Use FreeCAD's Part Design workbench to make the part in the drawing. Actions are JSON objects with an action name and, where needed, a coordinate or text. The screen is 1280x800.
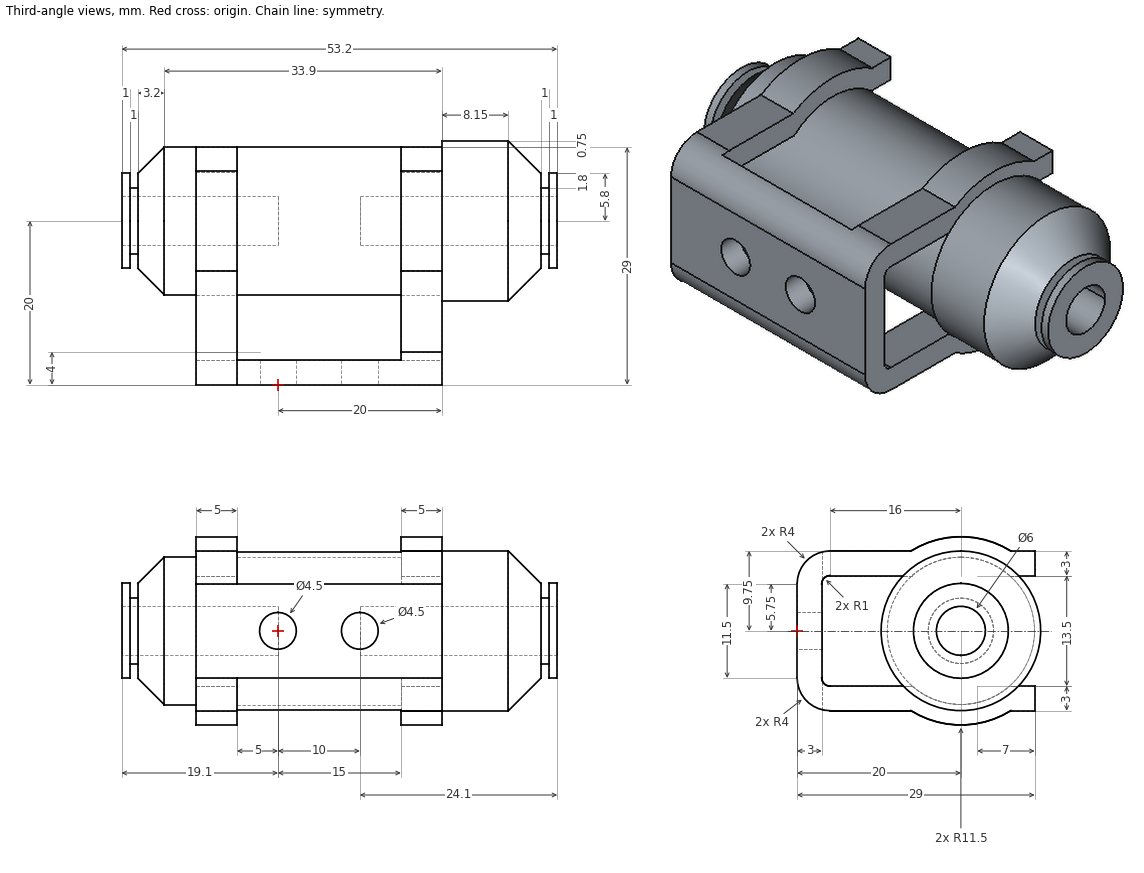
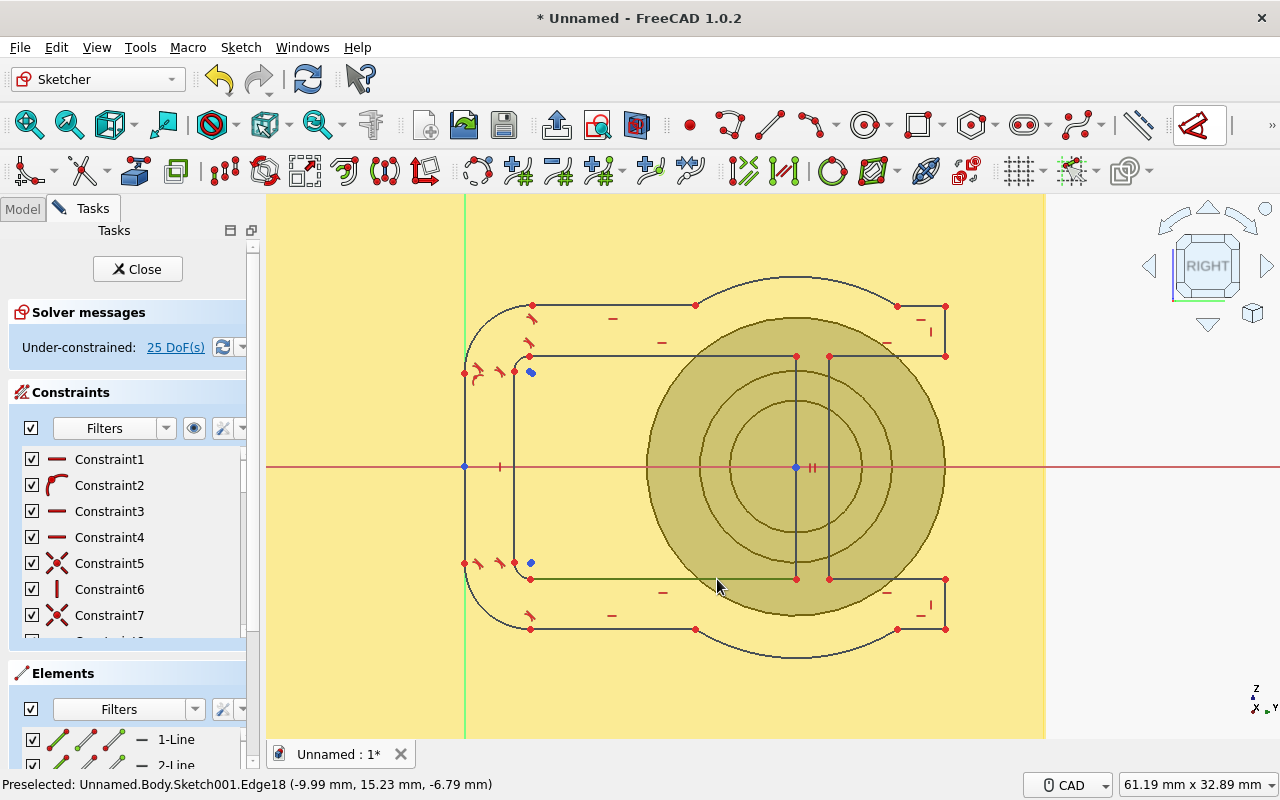
{"action": "left_click", "coordinate": [519, 574]}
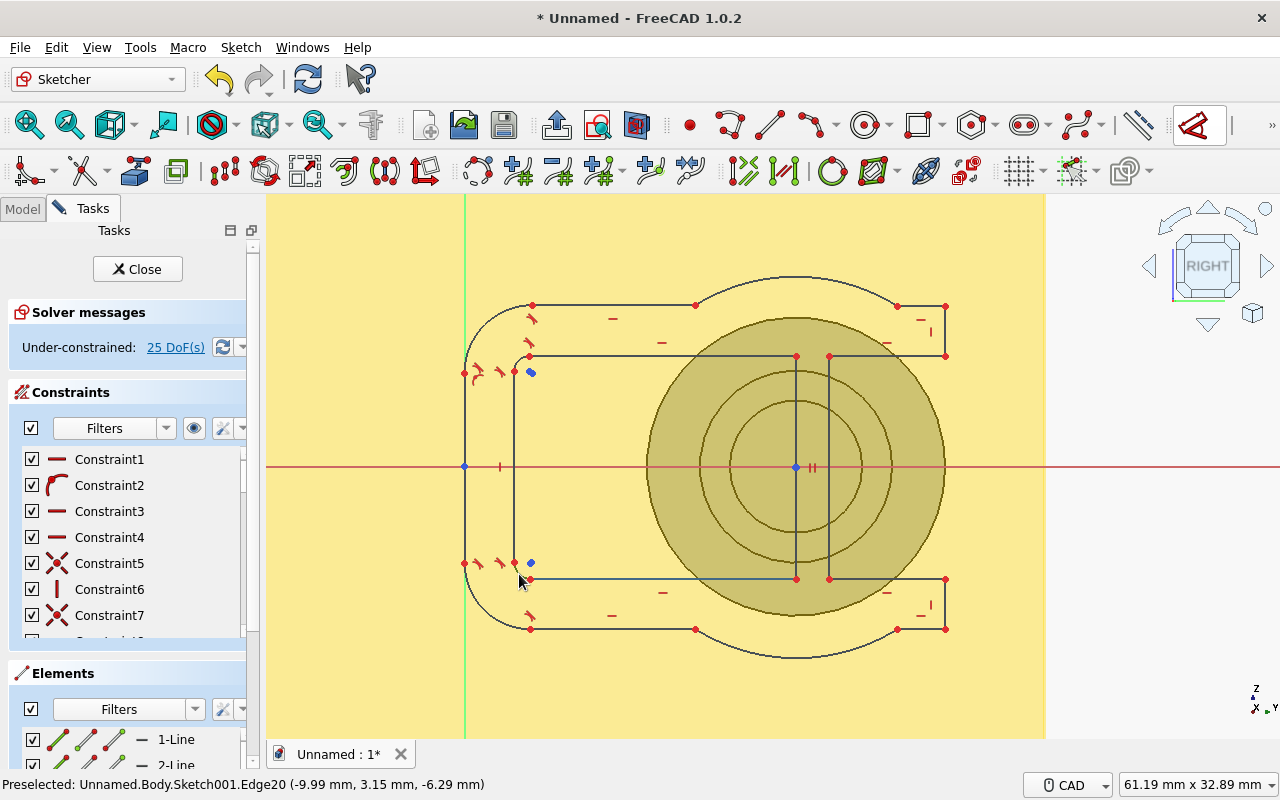
{"action": "key", "text": "t"}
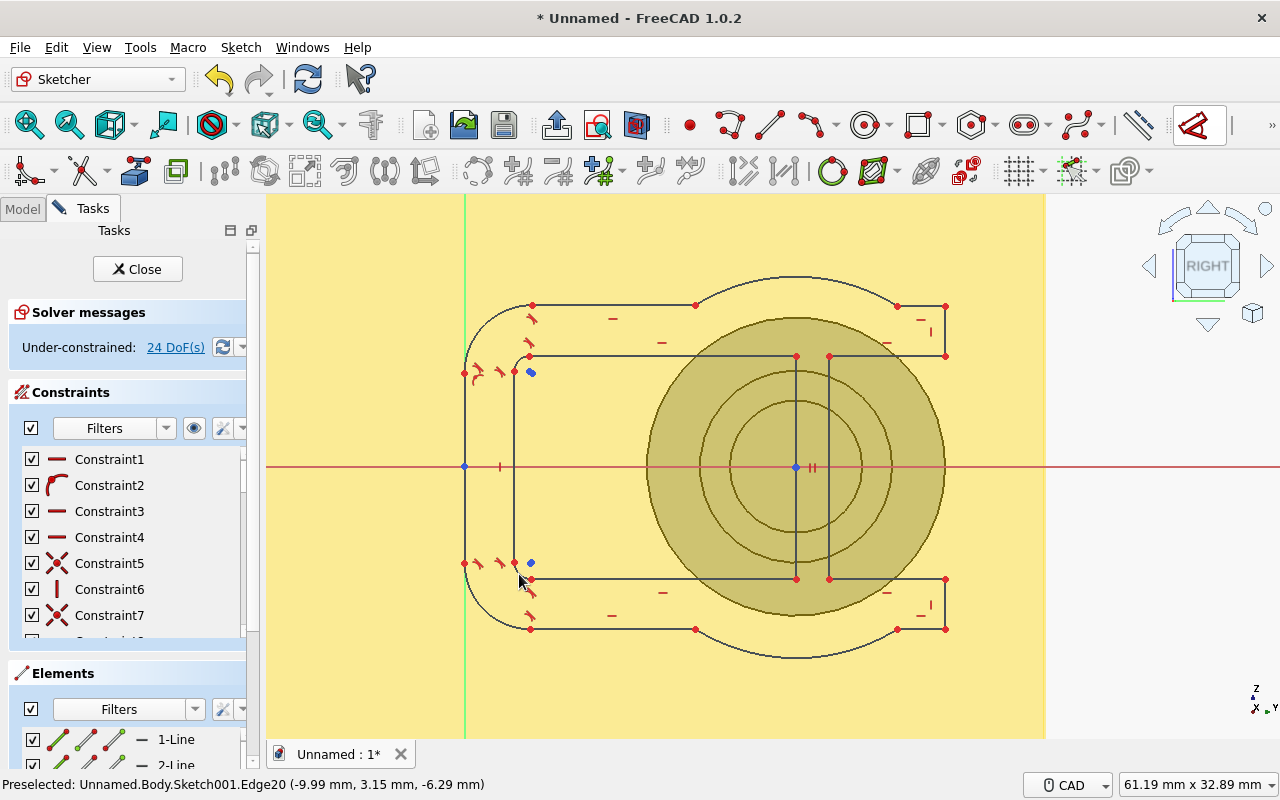
{"action": "left_click", "coordinate": [465, 430]}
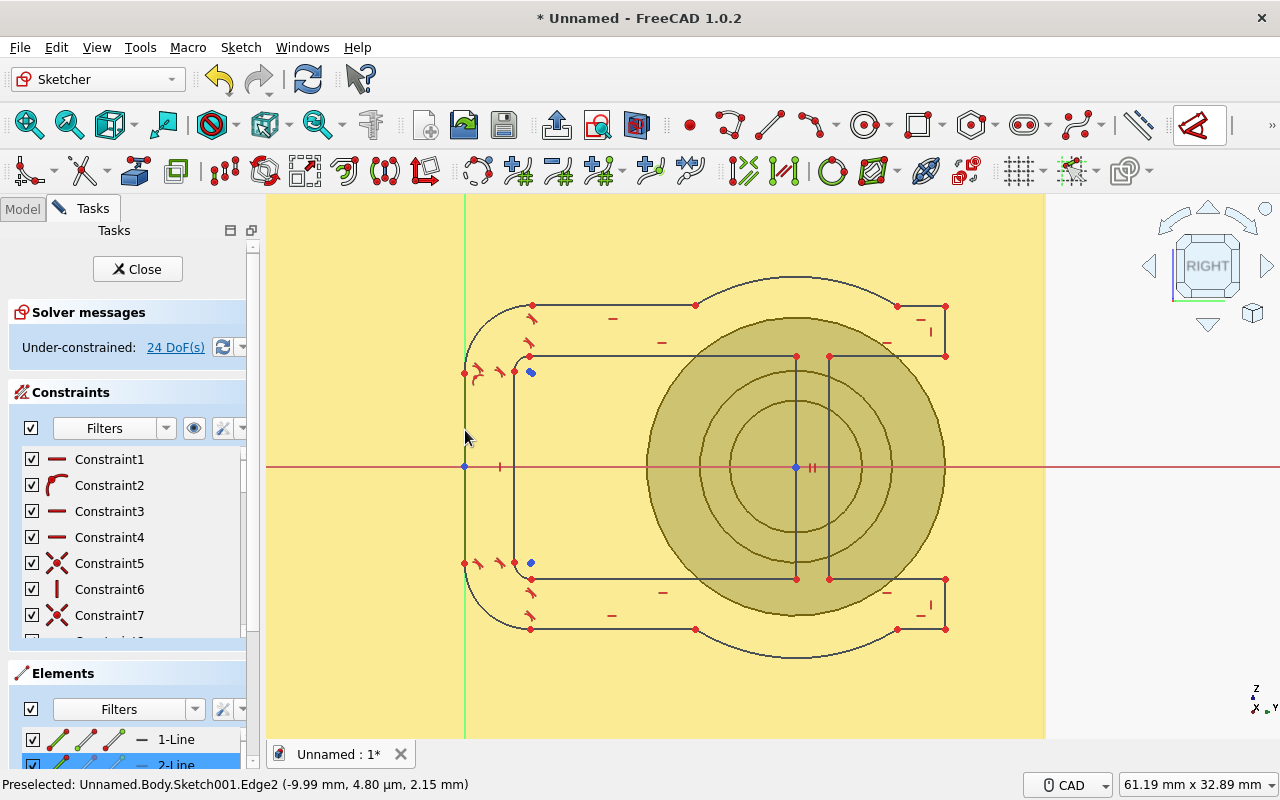
{"action": "key", "text": "v"}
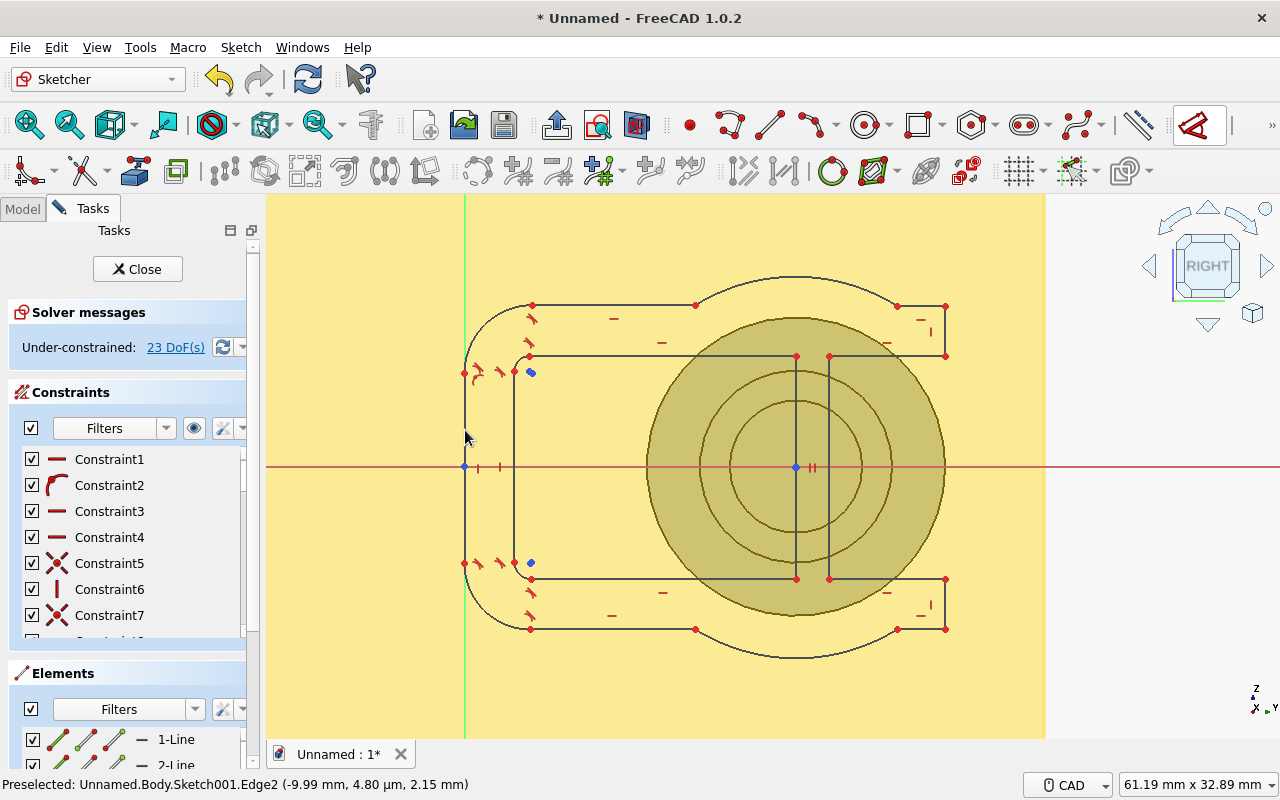
{"action": "left_click", "coordinate": [754, 654]}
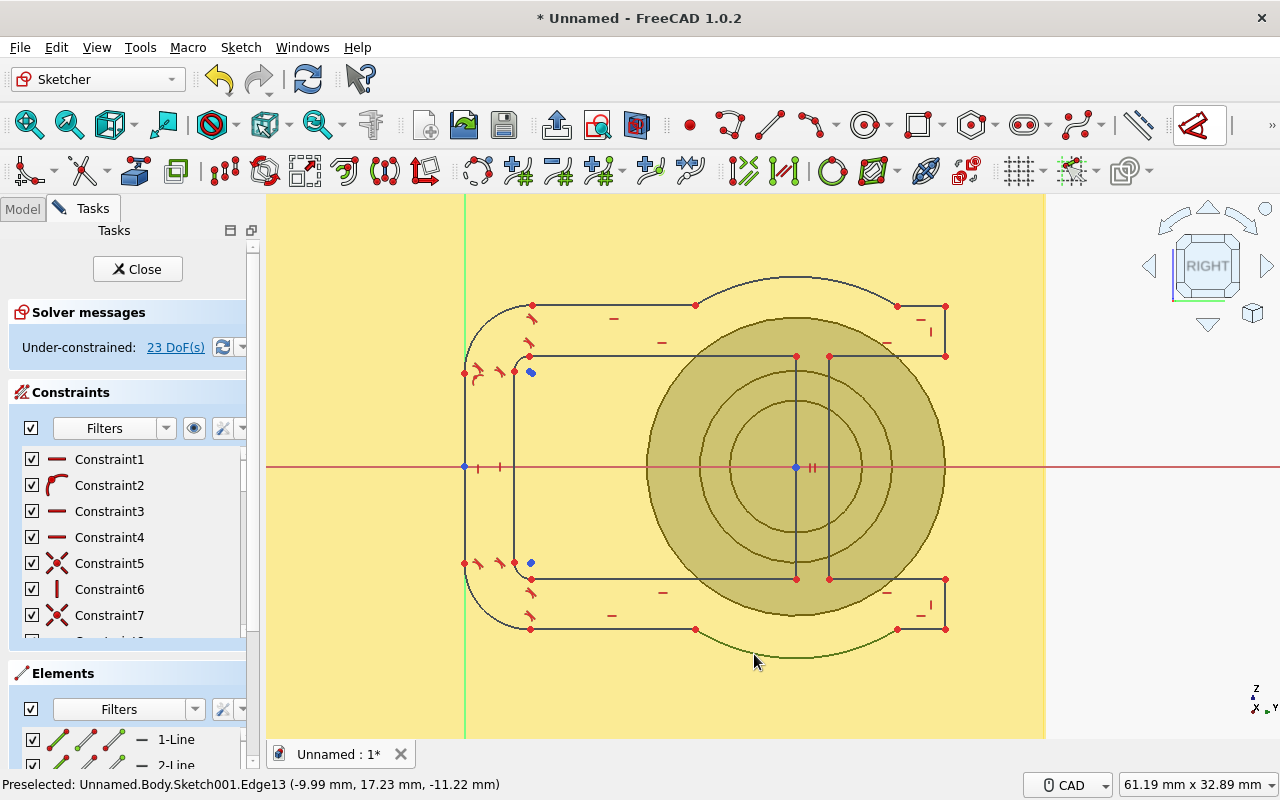
{"action": "left_click", "coordinate": [839, 282]}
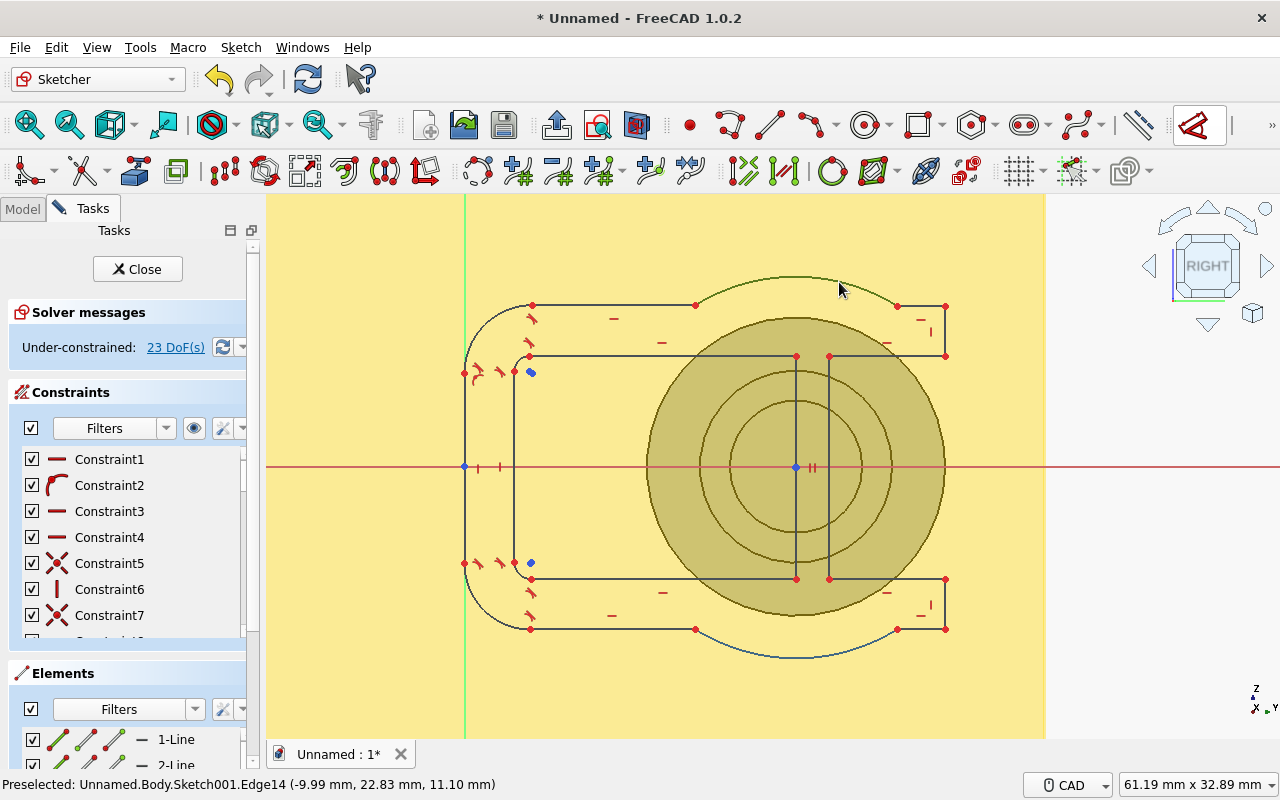
{"action": "key", "text": "c"}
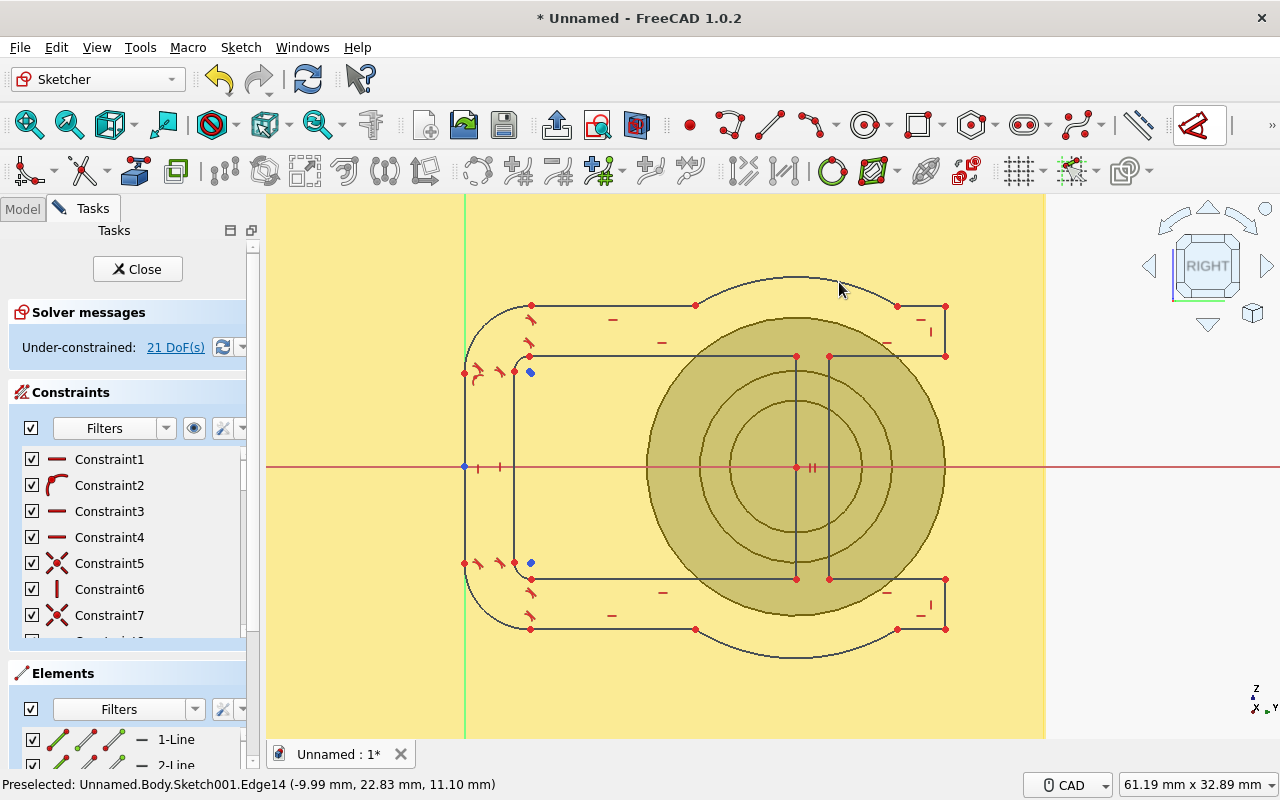
{"action": "left_click", "coordinate": [501, 313]}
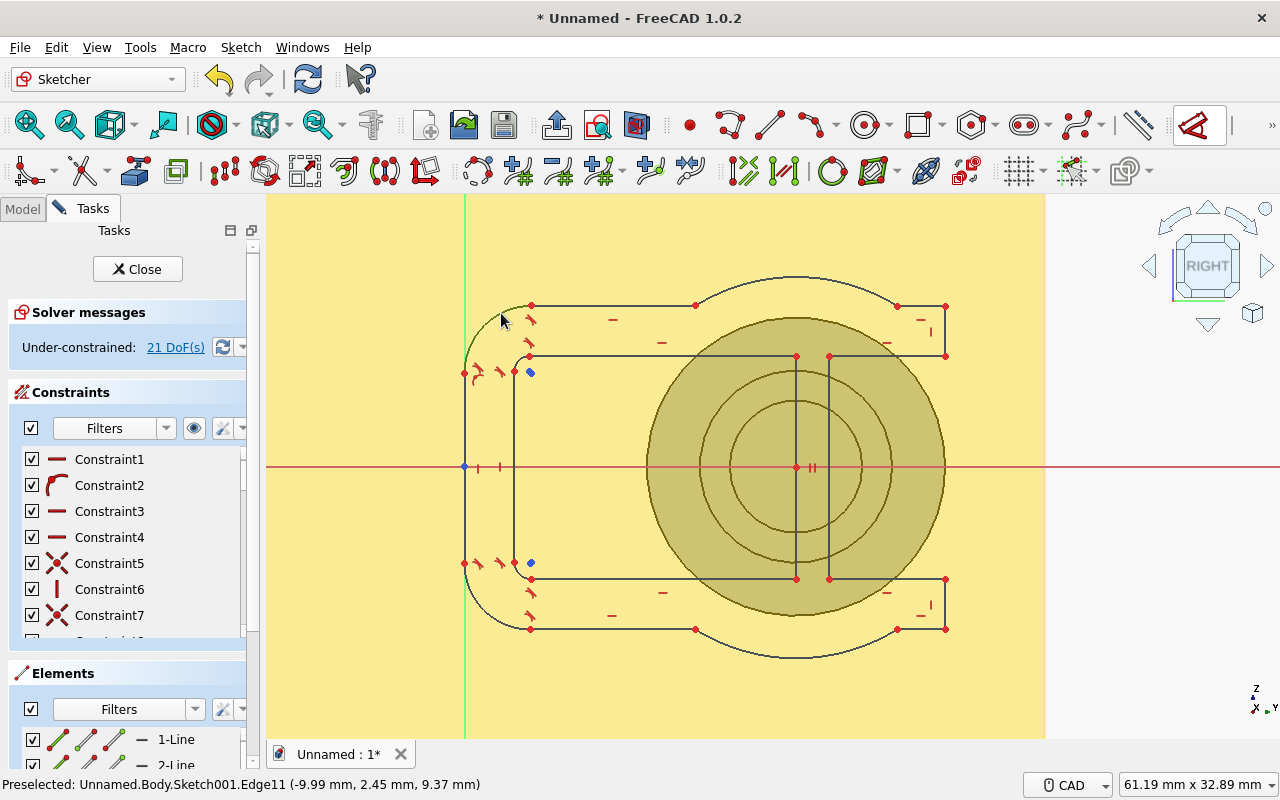
{"action": "left_click", "coordinate": [519, 361]}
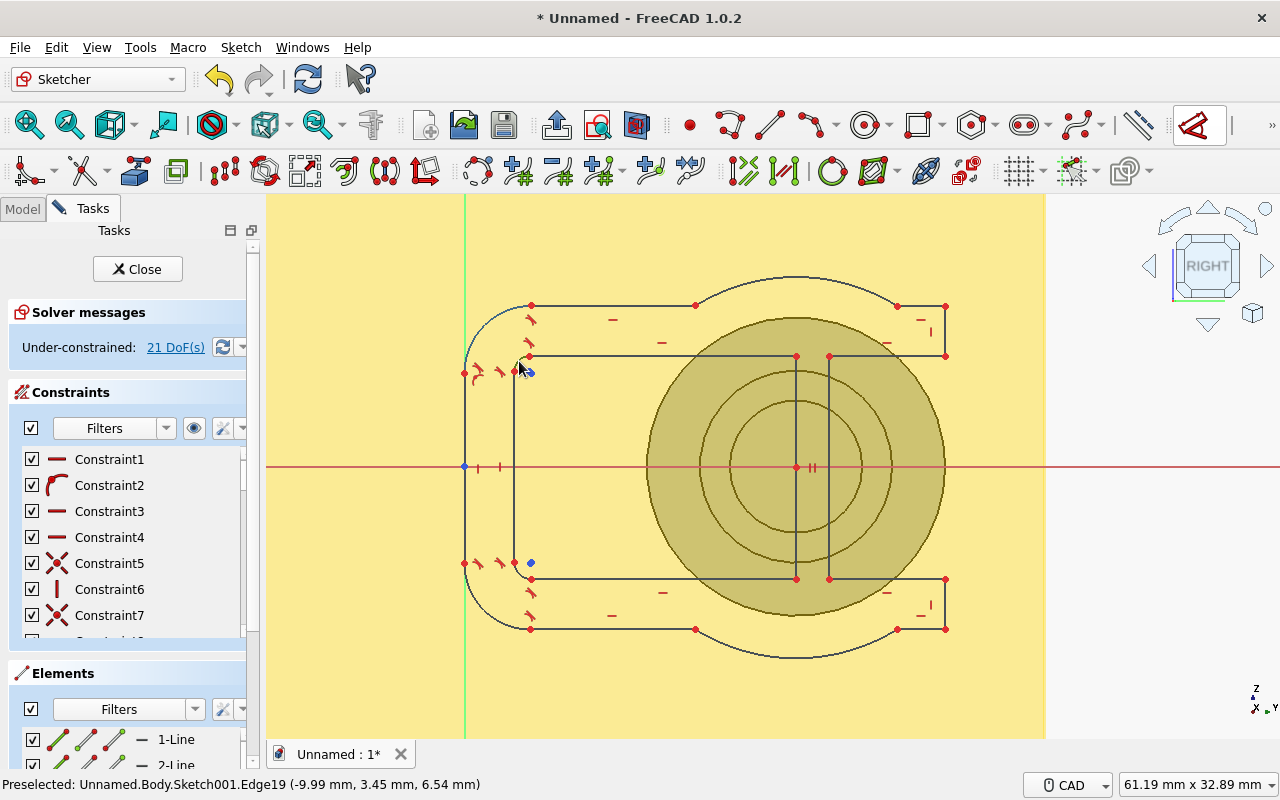
{"action": "key", "text": "c"}